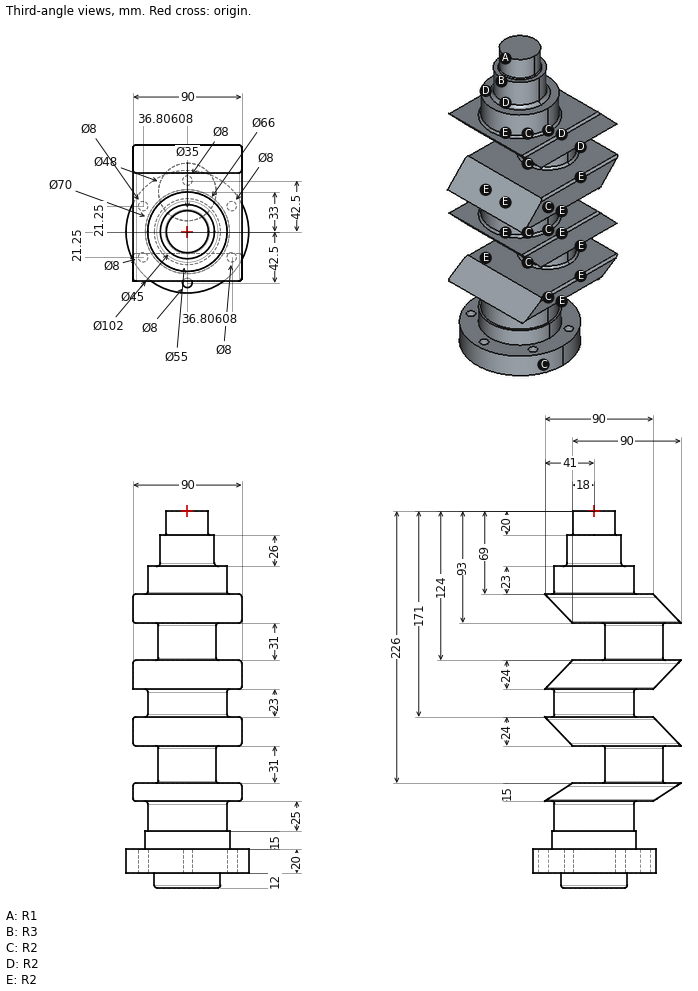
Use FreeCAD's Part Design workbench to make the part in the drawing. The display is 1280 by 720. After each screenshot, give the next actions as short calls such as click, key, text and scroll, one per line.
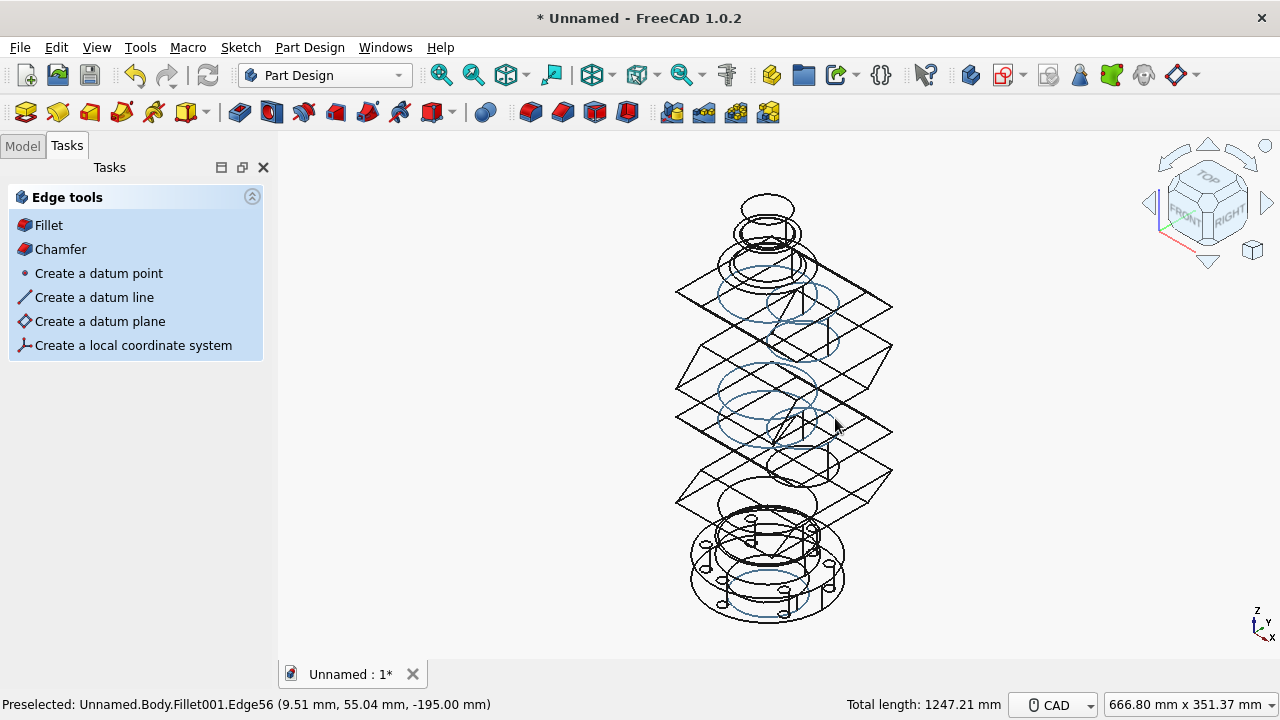
click(835, 456, ctrl)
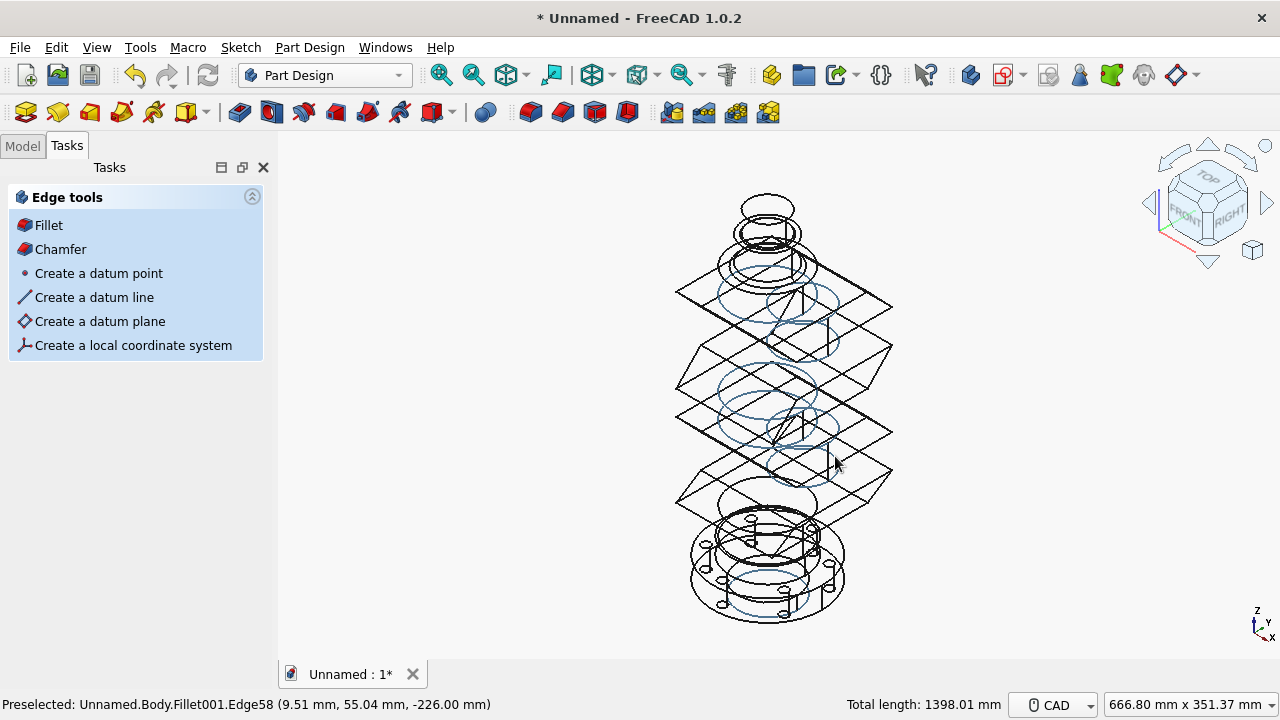
click(719, 500, ctrl)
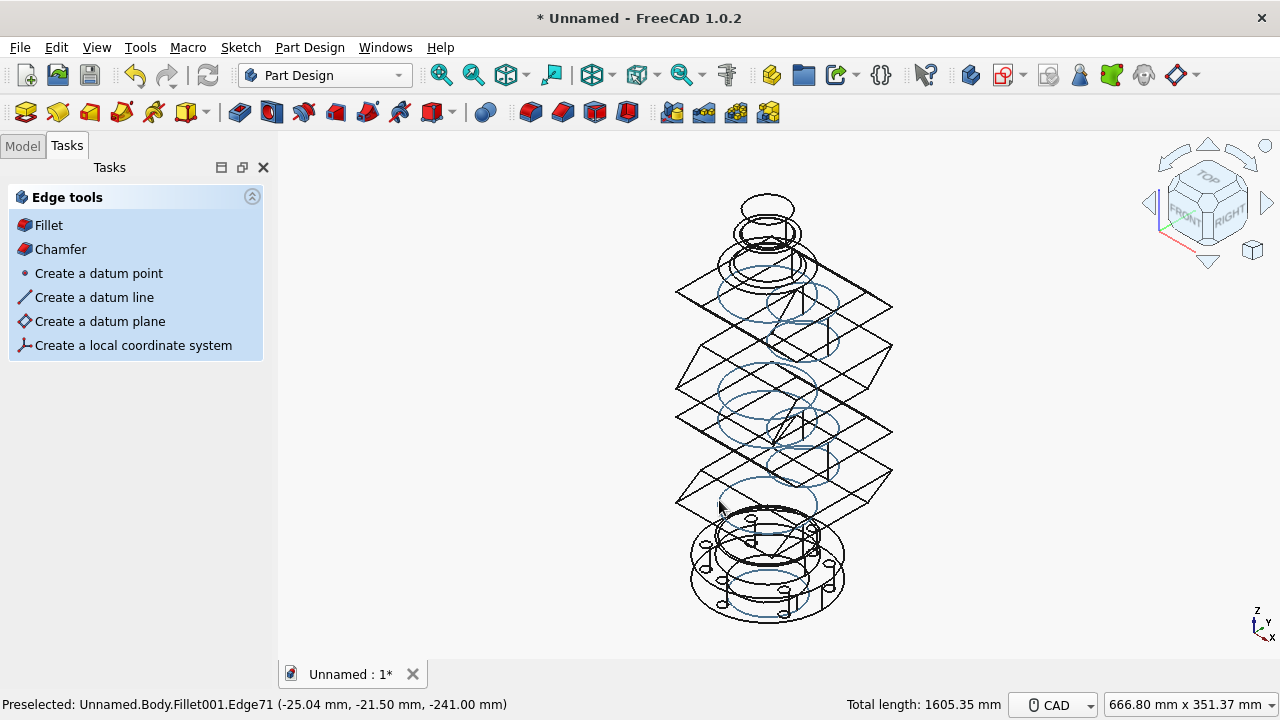
key(v)
key(1)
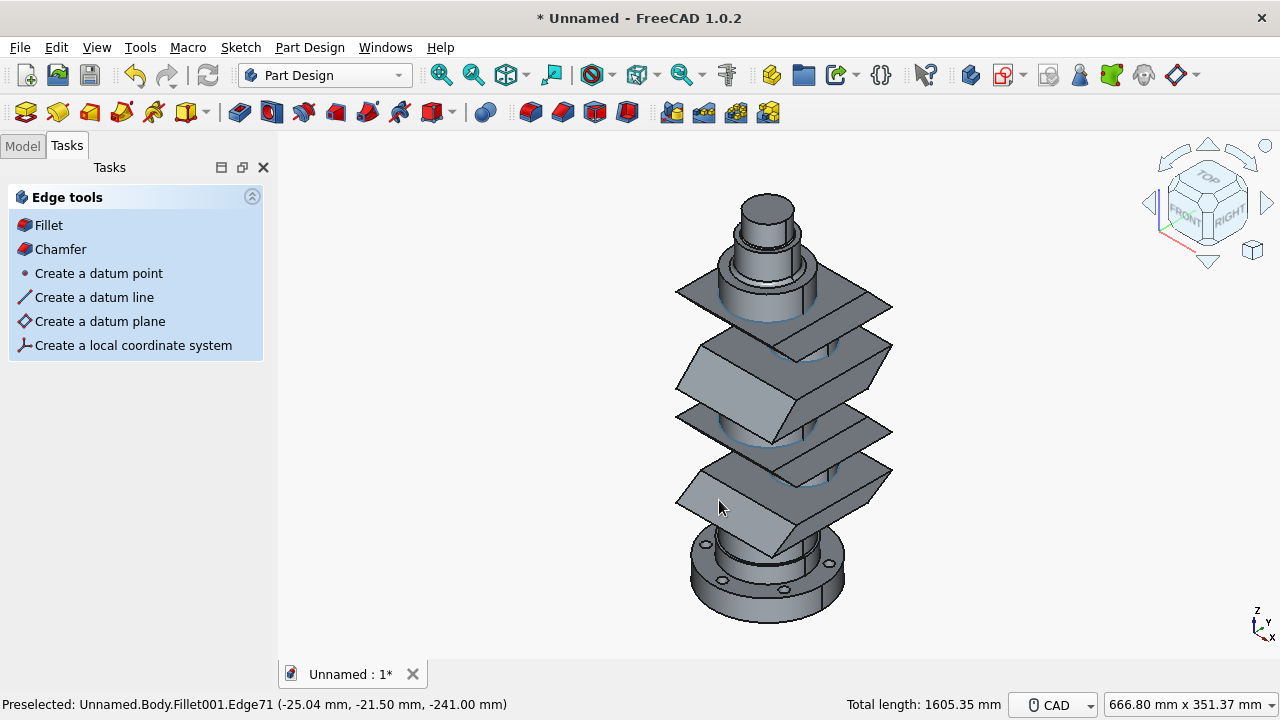
click(532, 112)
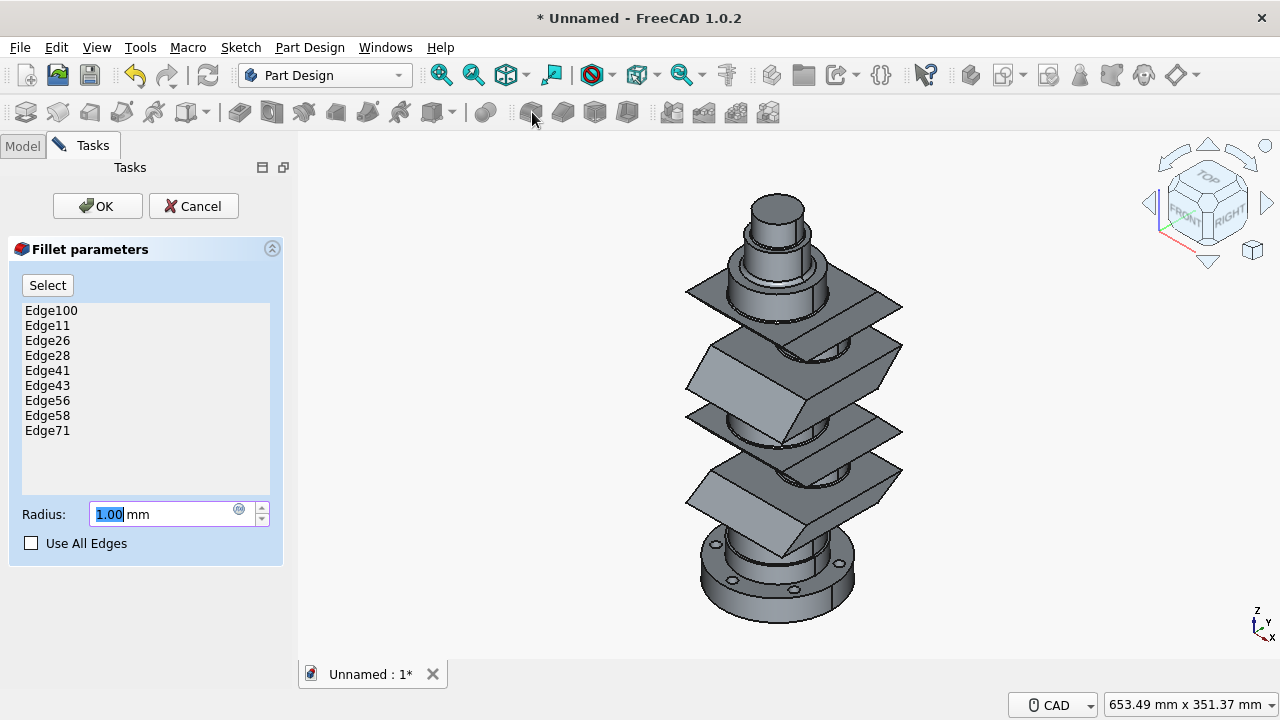
text(2)
key(Tab)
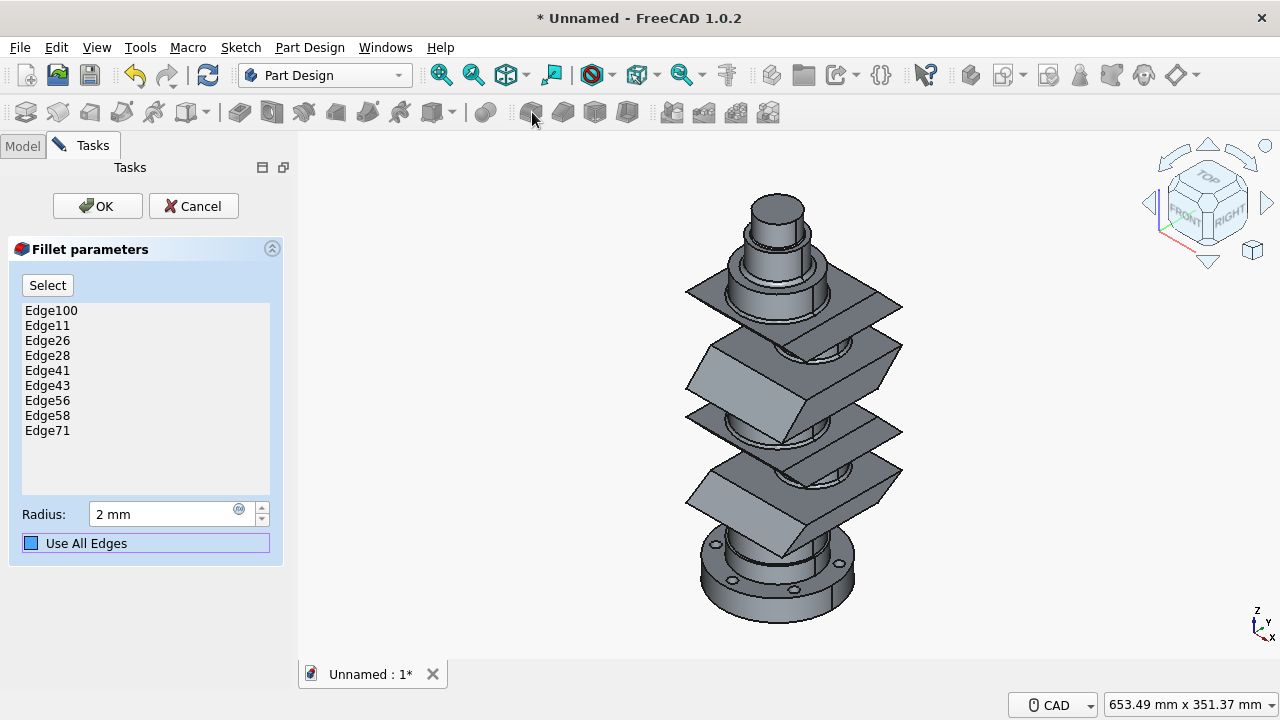
click(98, 206)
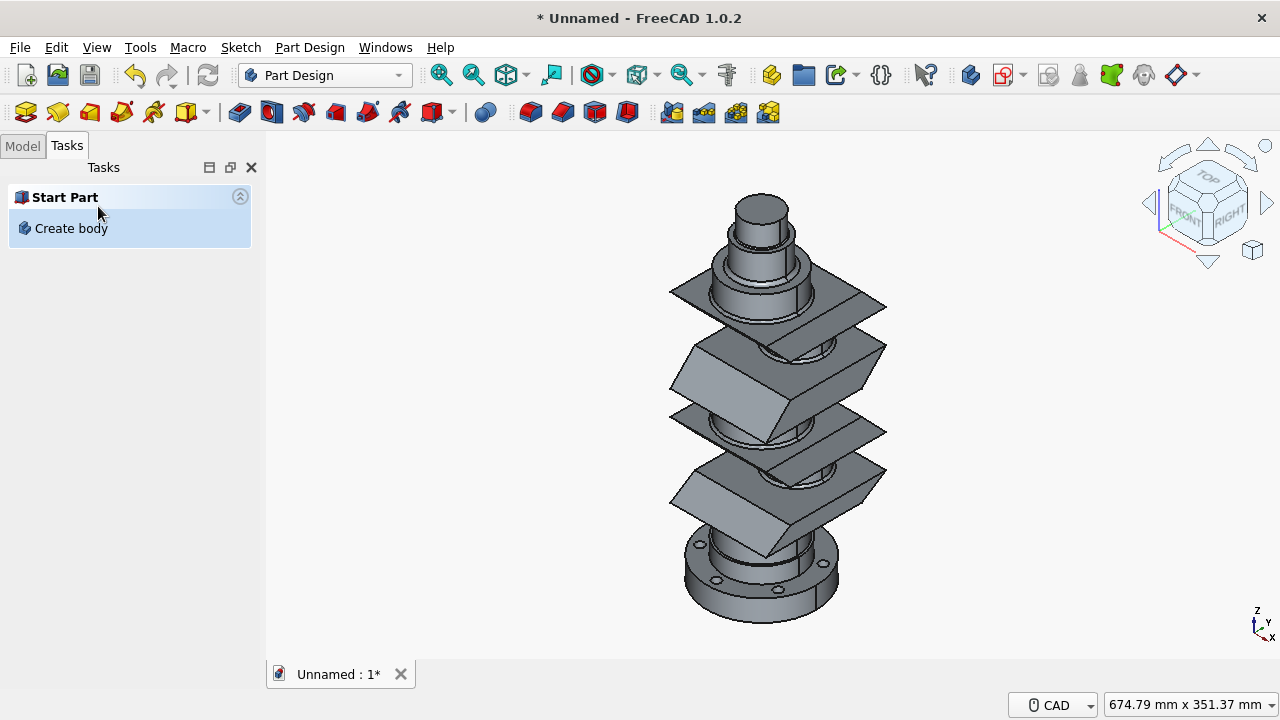
click(814, 318)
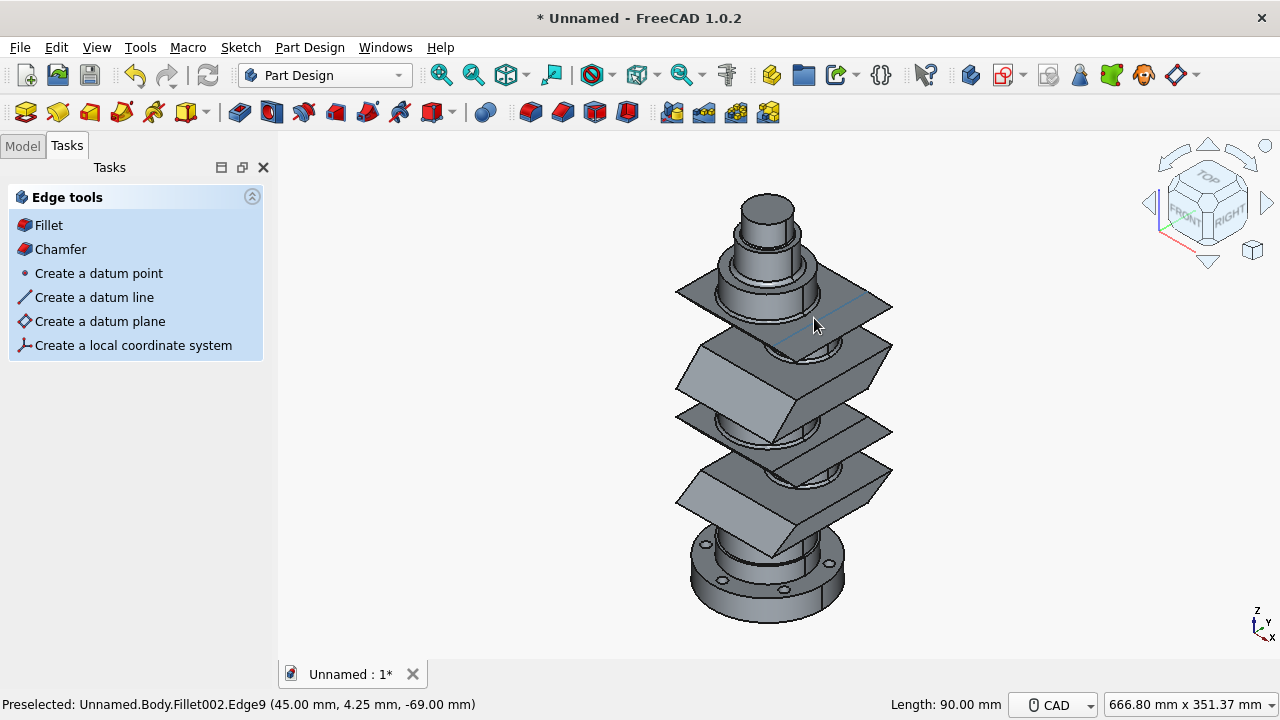
key(2)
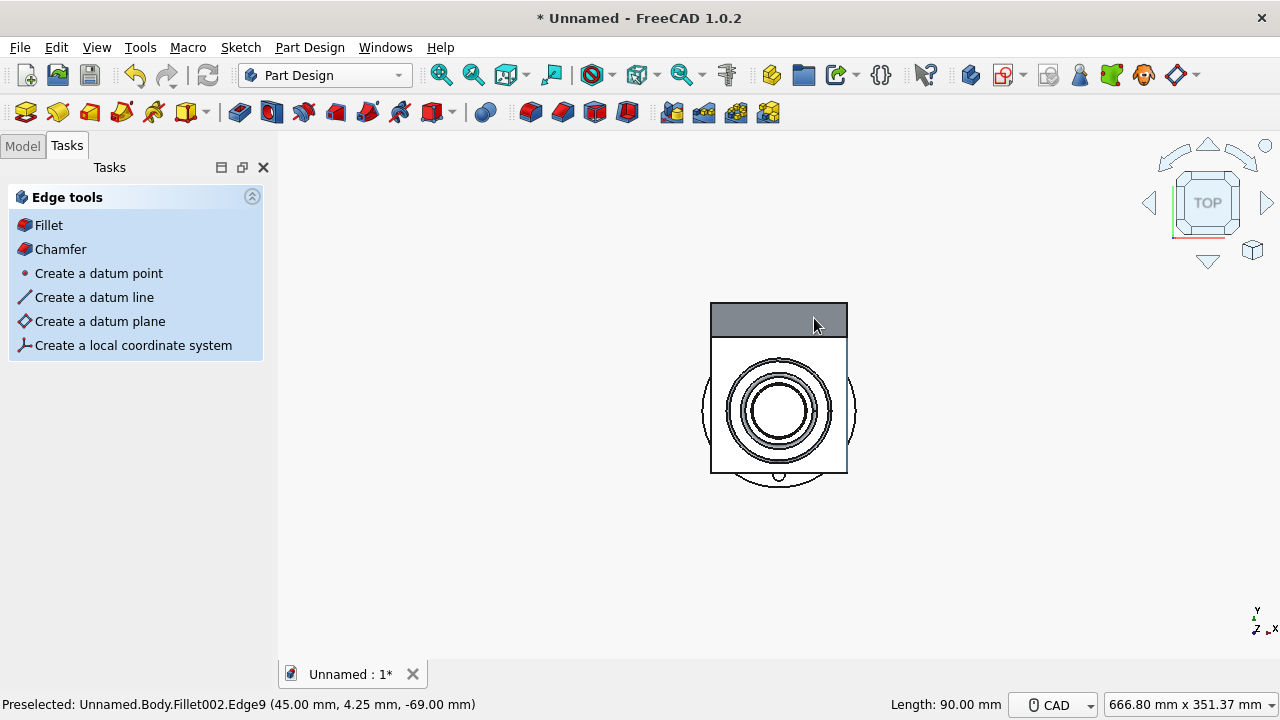
click(442, 76)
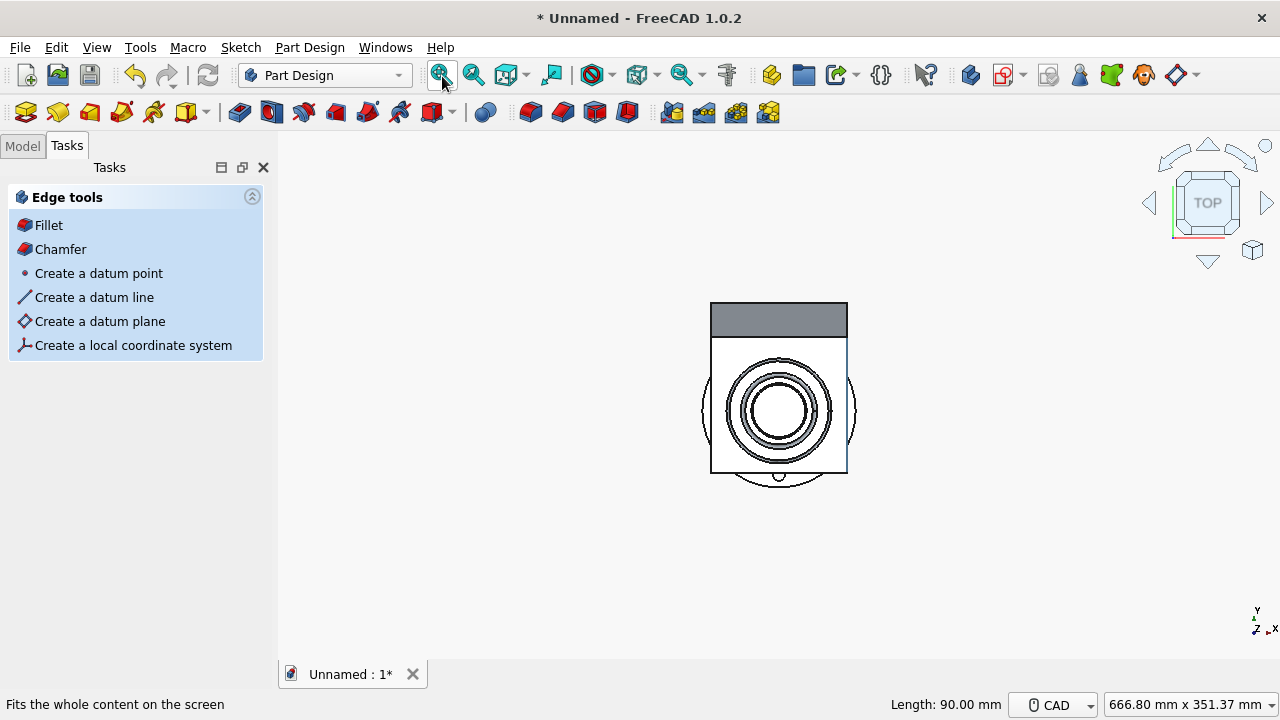
click(711, 404, ctrl)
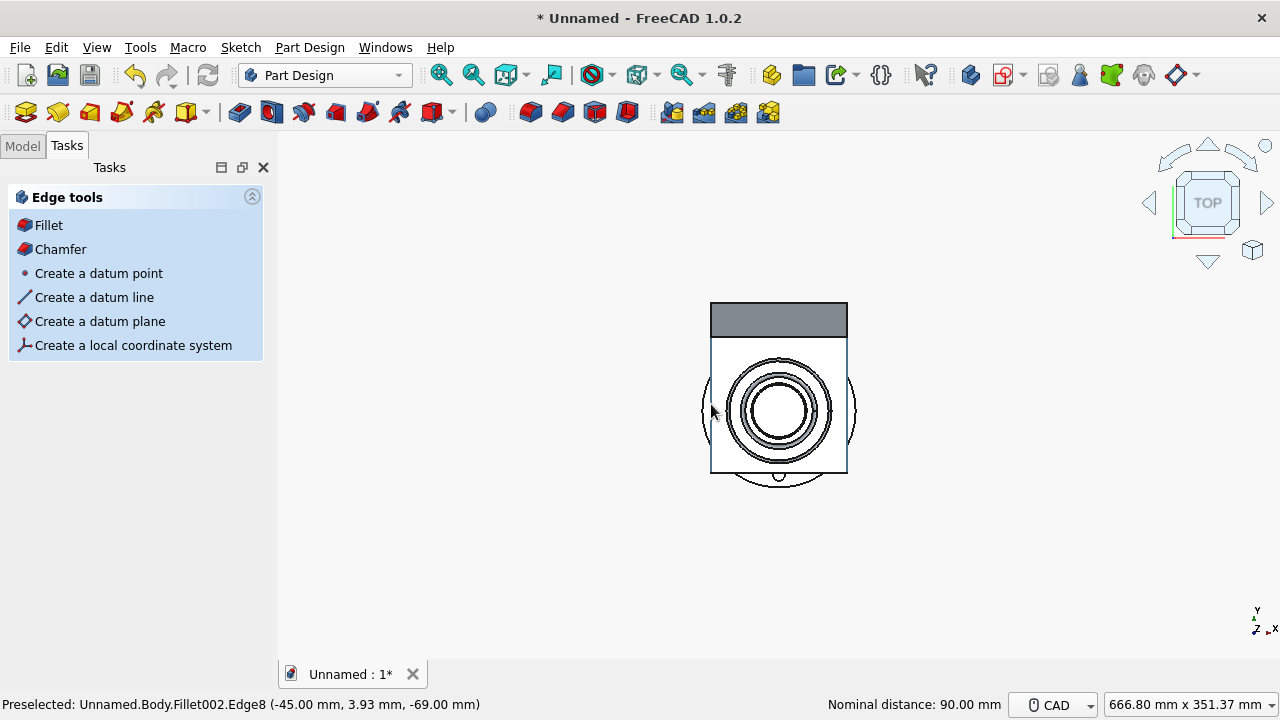
key(0)